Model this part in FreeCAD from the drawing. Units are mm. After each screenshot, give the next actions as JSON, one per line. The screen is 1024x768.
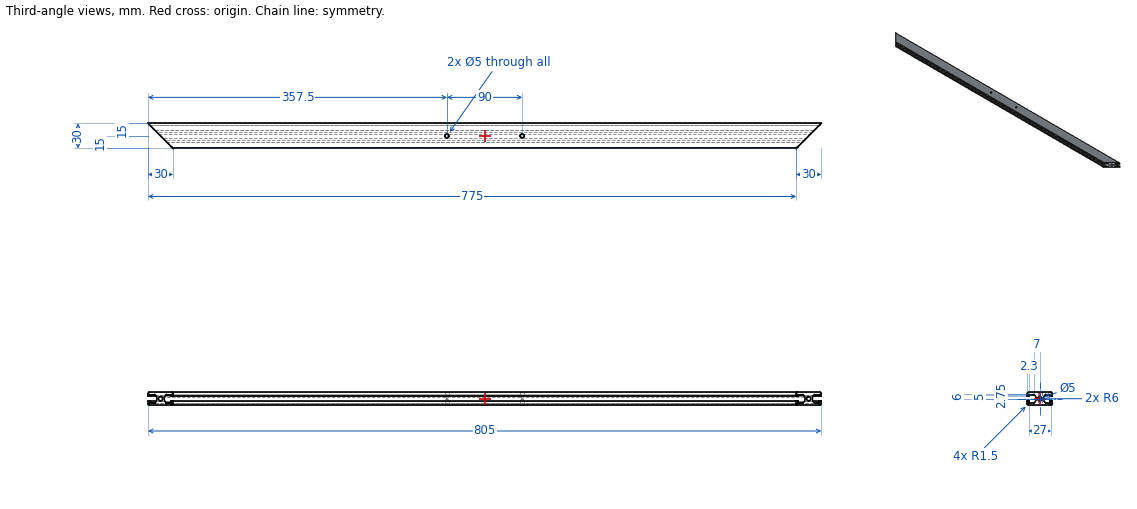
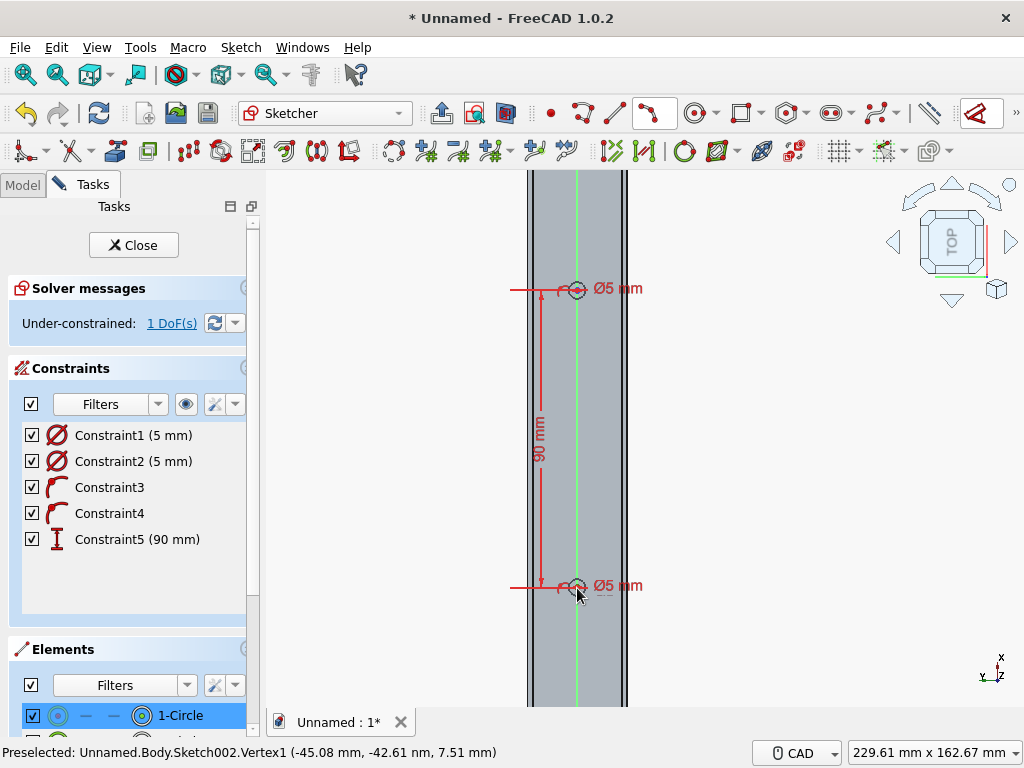
{"action": "key", "text": "i"}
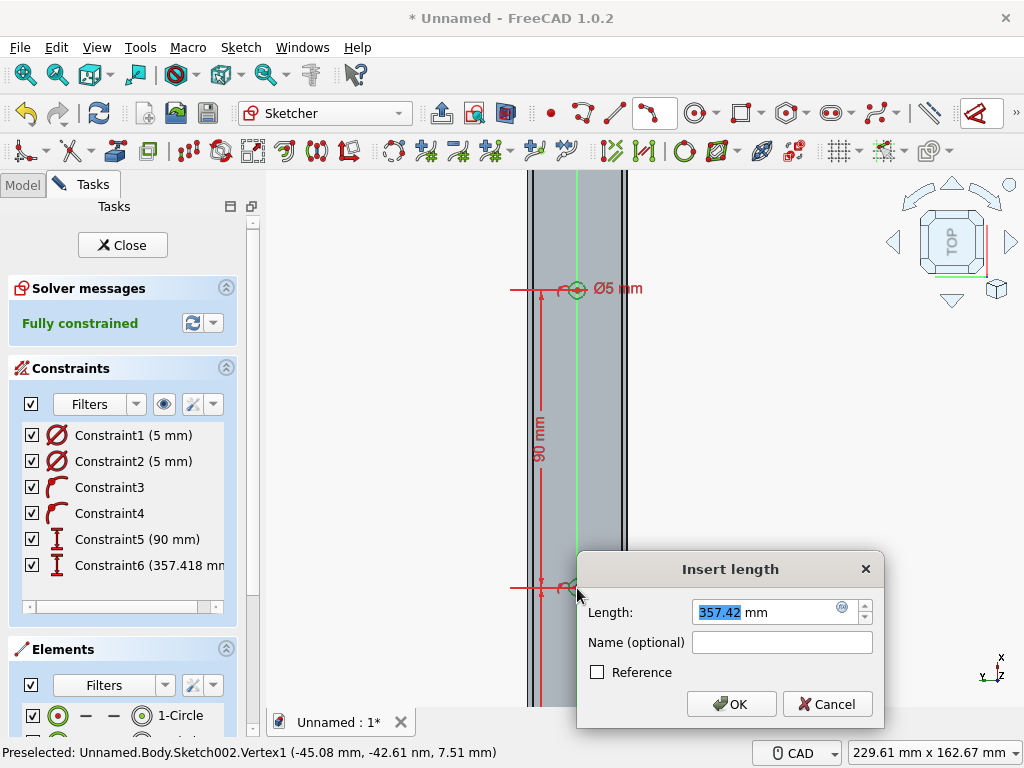
{"action": "type", "text": "357.5"}
{"action": "key", "text": "Return"}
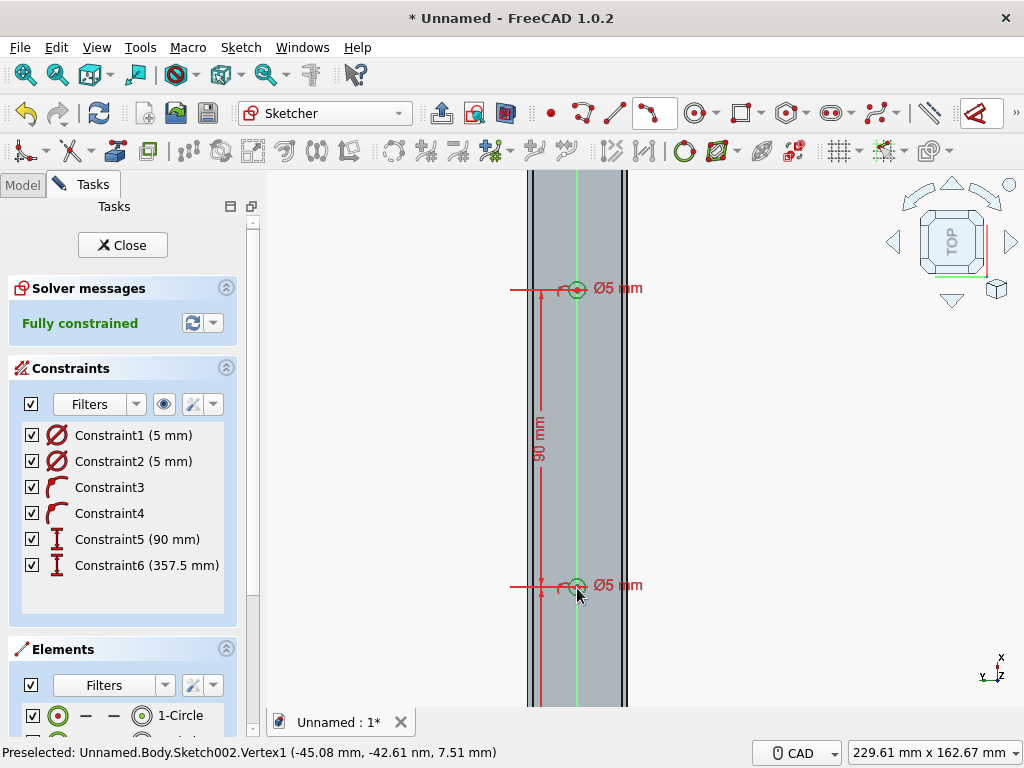
{"action": "left_click", "coordinate": [123, 245]}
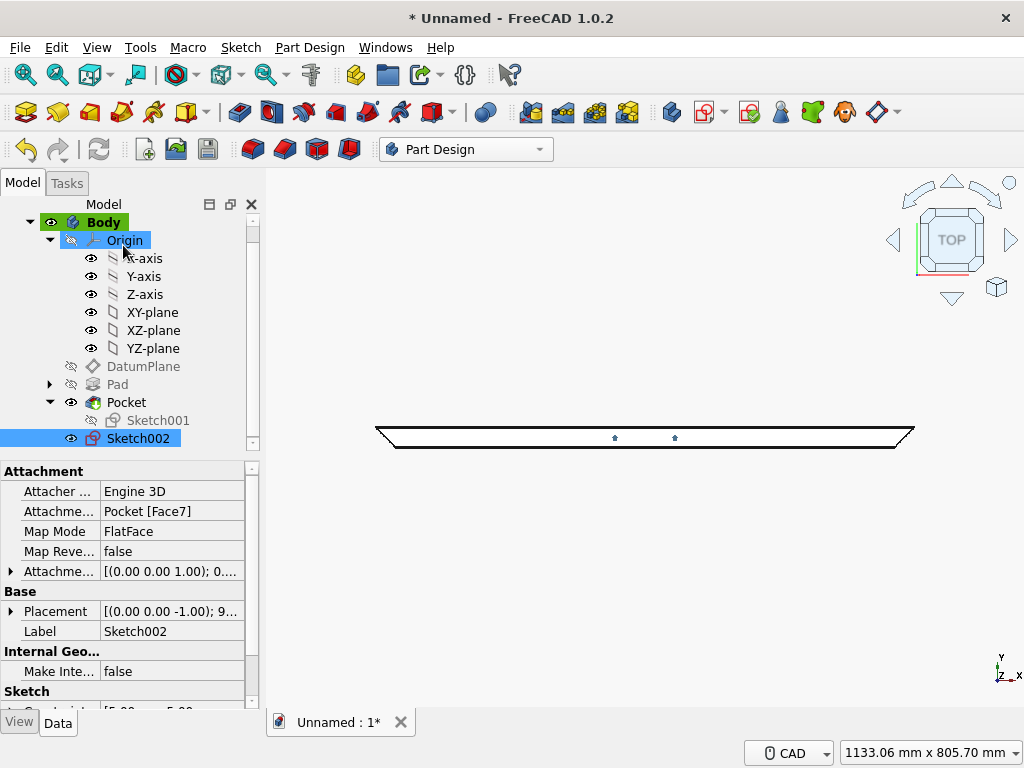
{"action": "left_click", "coordinate": [272, 112]}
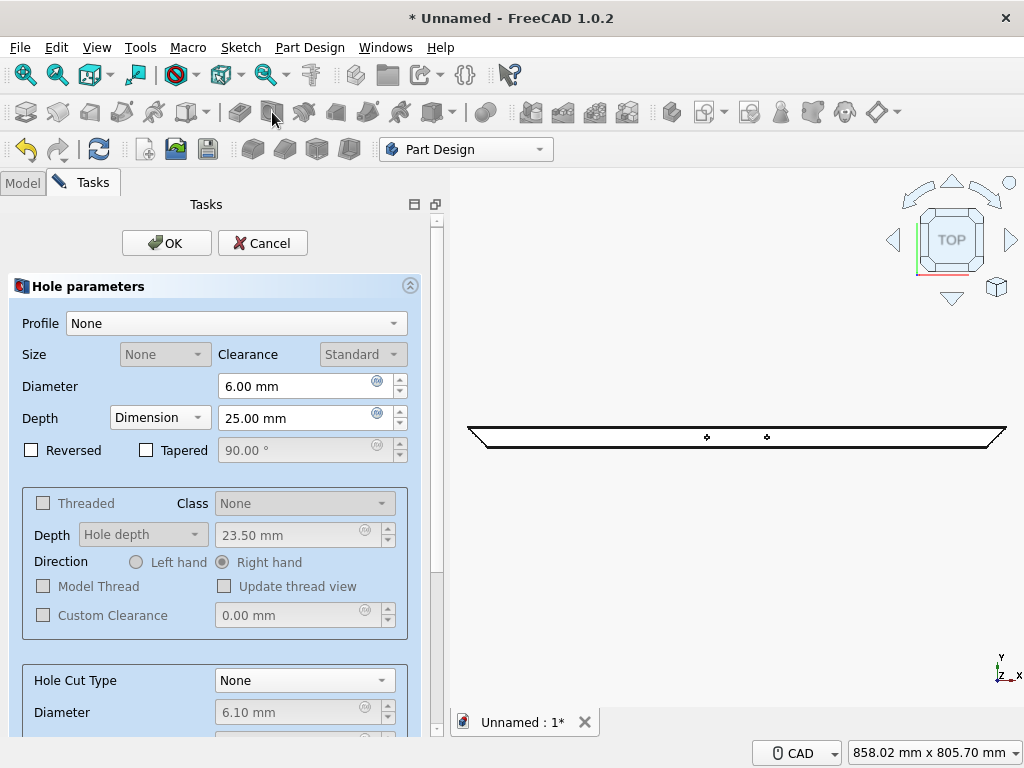
{"action": "triple_click", "coordinate": [305, 386]}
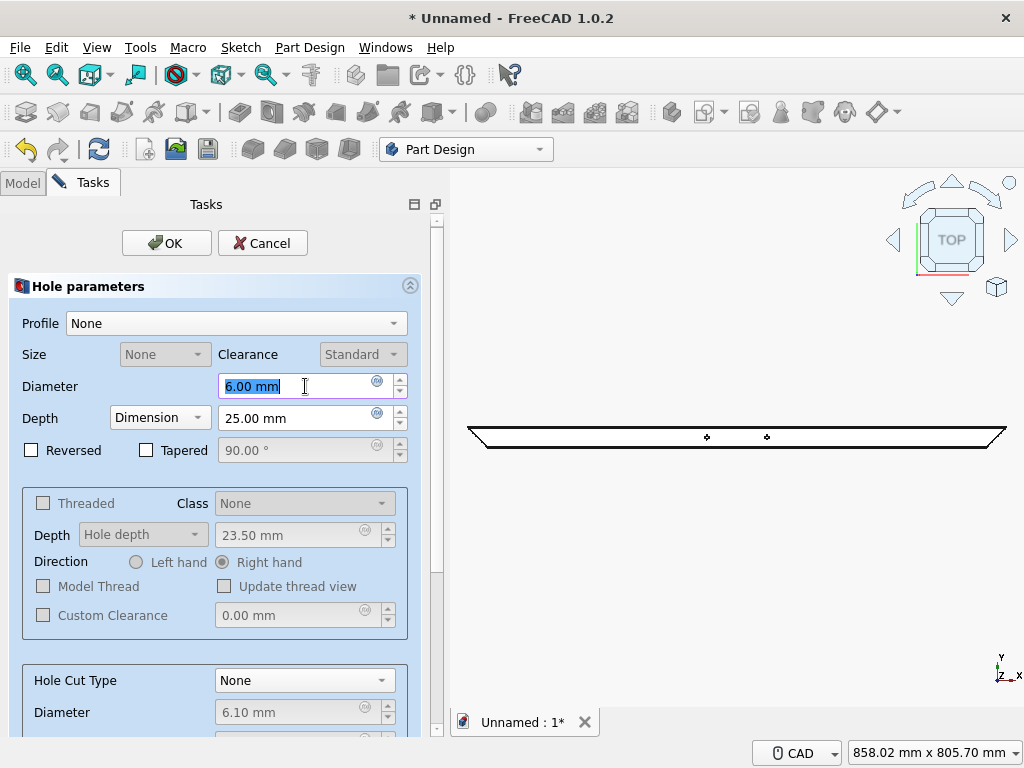
{"action": "type", "text": "5"}
{"action": "key", "text": "Tab"}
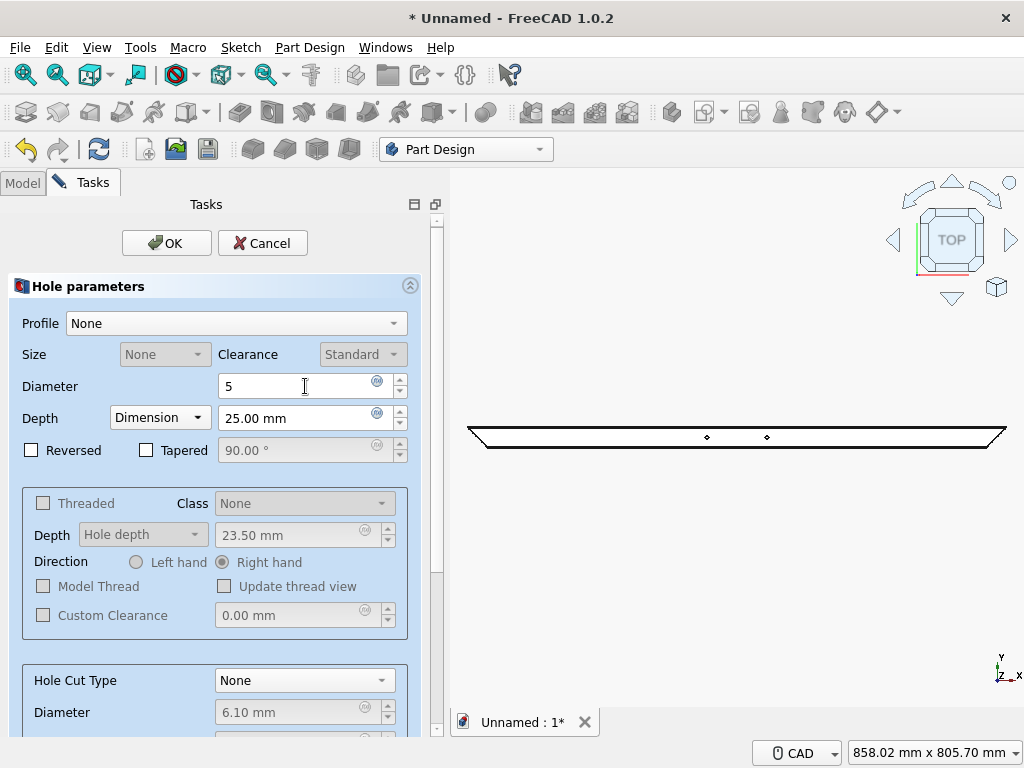
{"action": "left_click", "coordinate": [161, 418]}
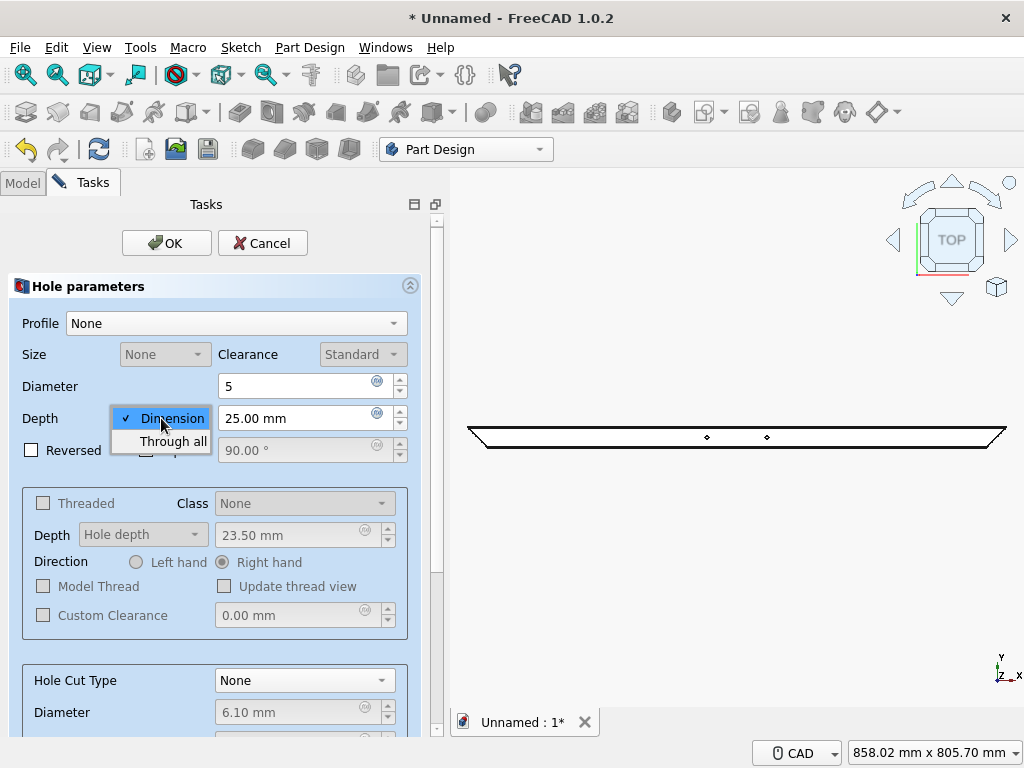
{"action": "left_click", "coordinate": [160, 442]}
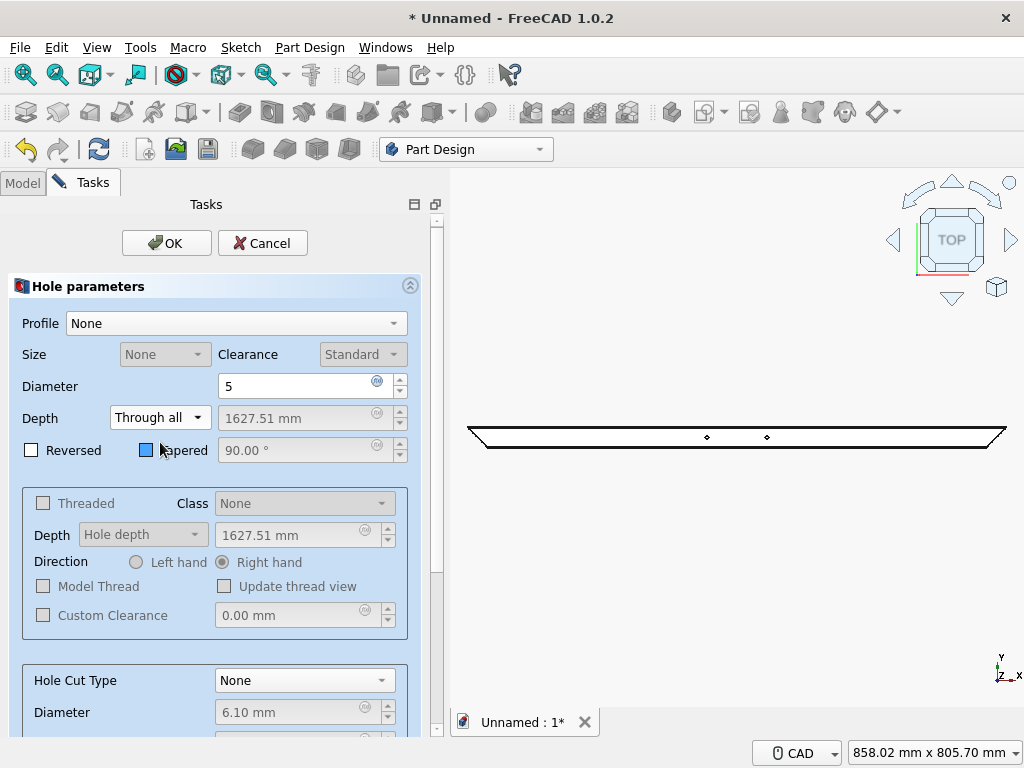
{"action": "left_click", "coordinate": [167, 243]}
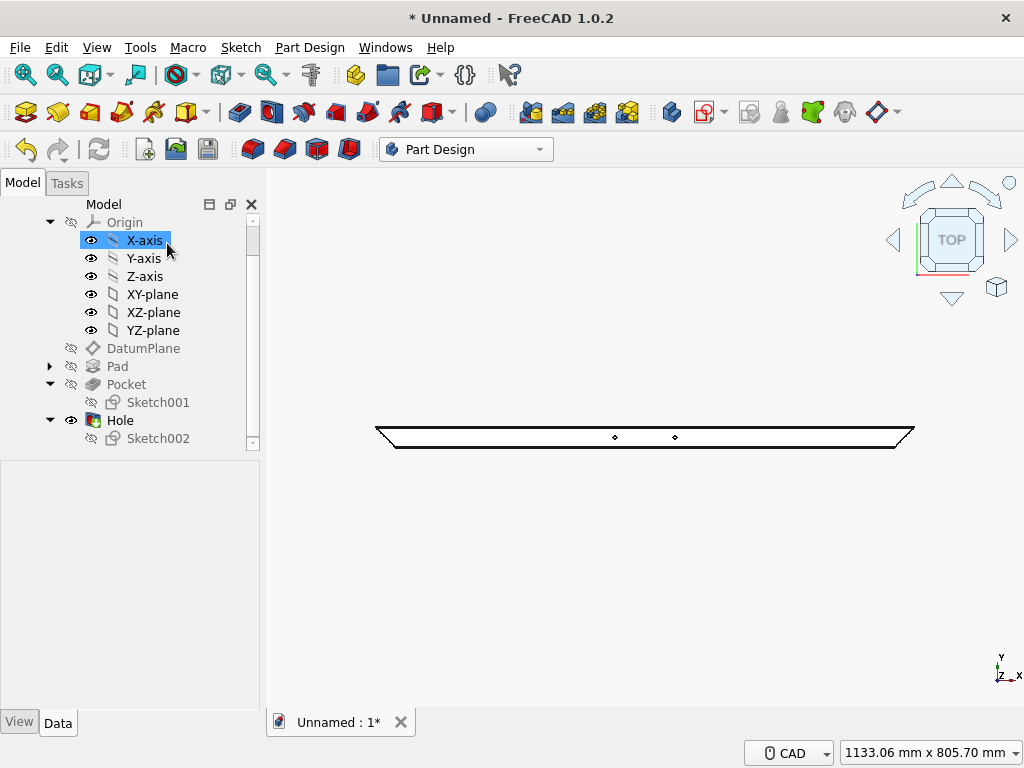
{"action": "key", "text": "0"}